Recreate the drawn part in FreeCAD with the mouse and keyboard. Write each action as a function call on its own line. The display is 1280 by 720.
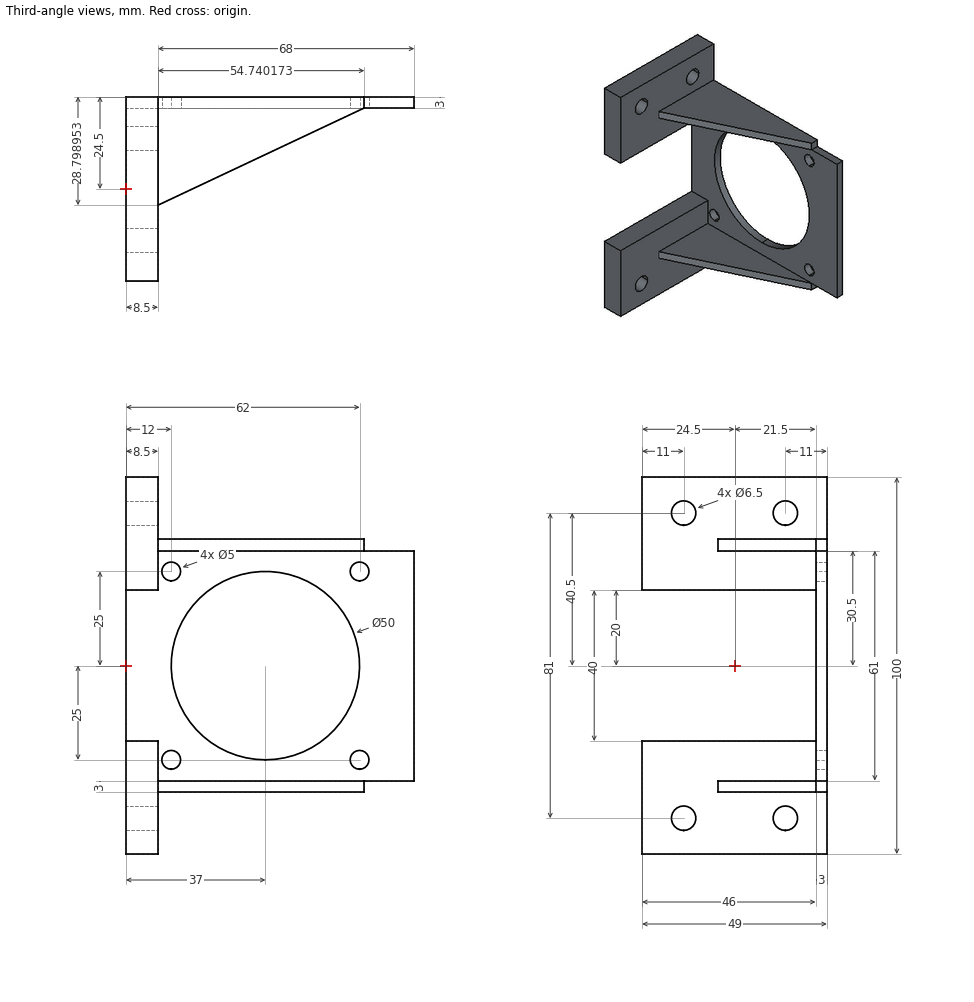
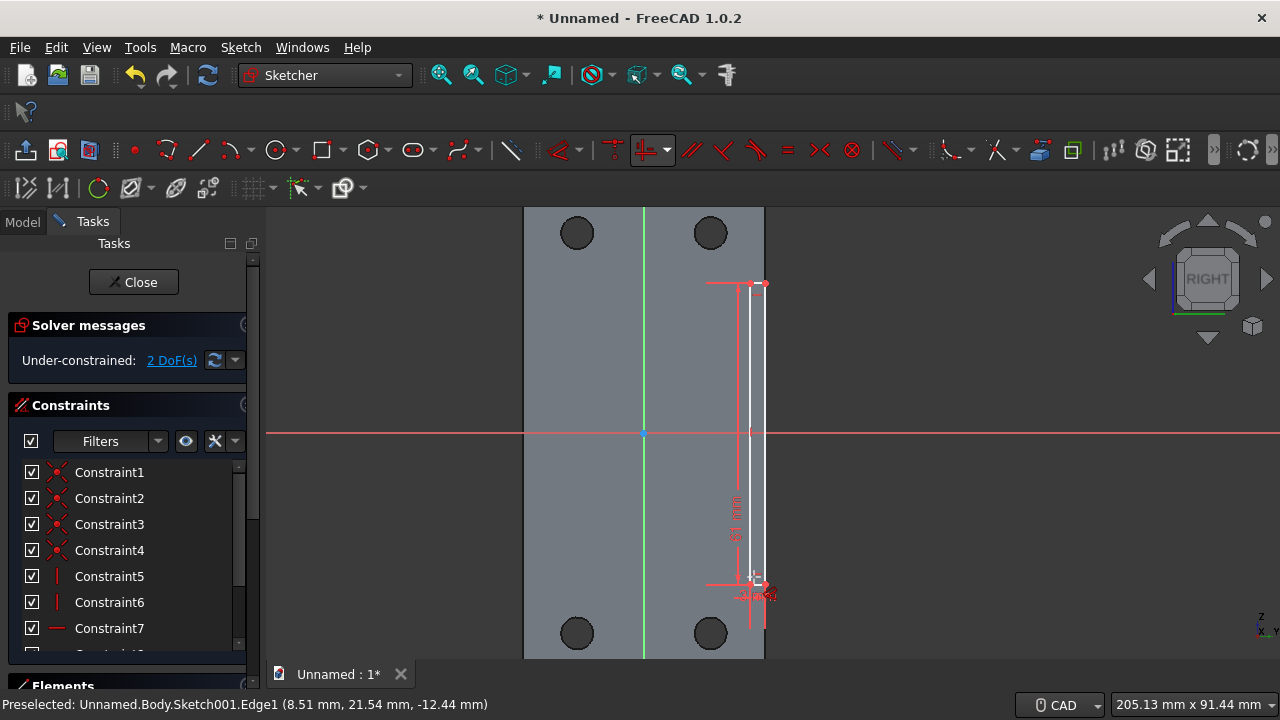
click(750, 283)
click(697, 249)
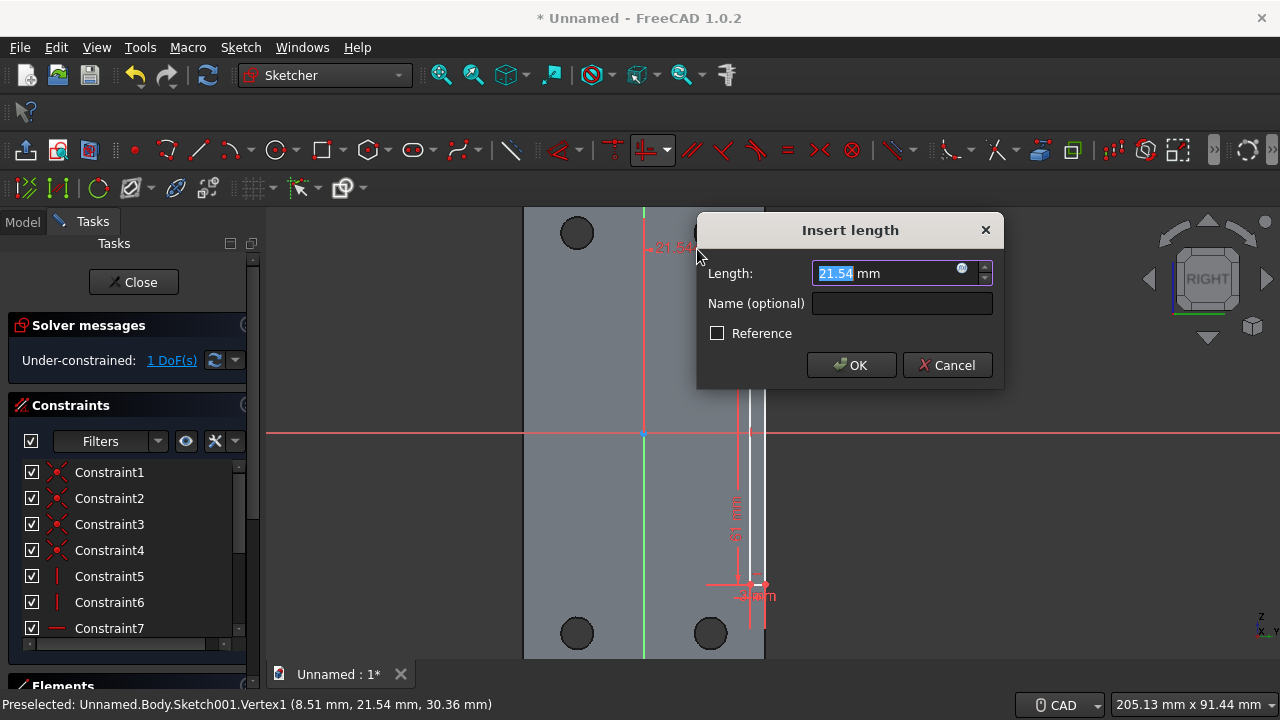
text(21.5)
key(Return)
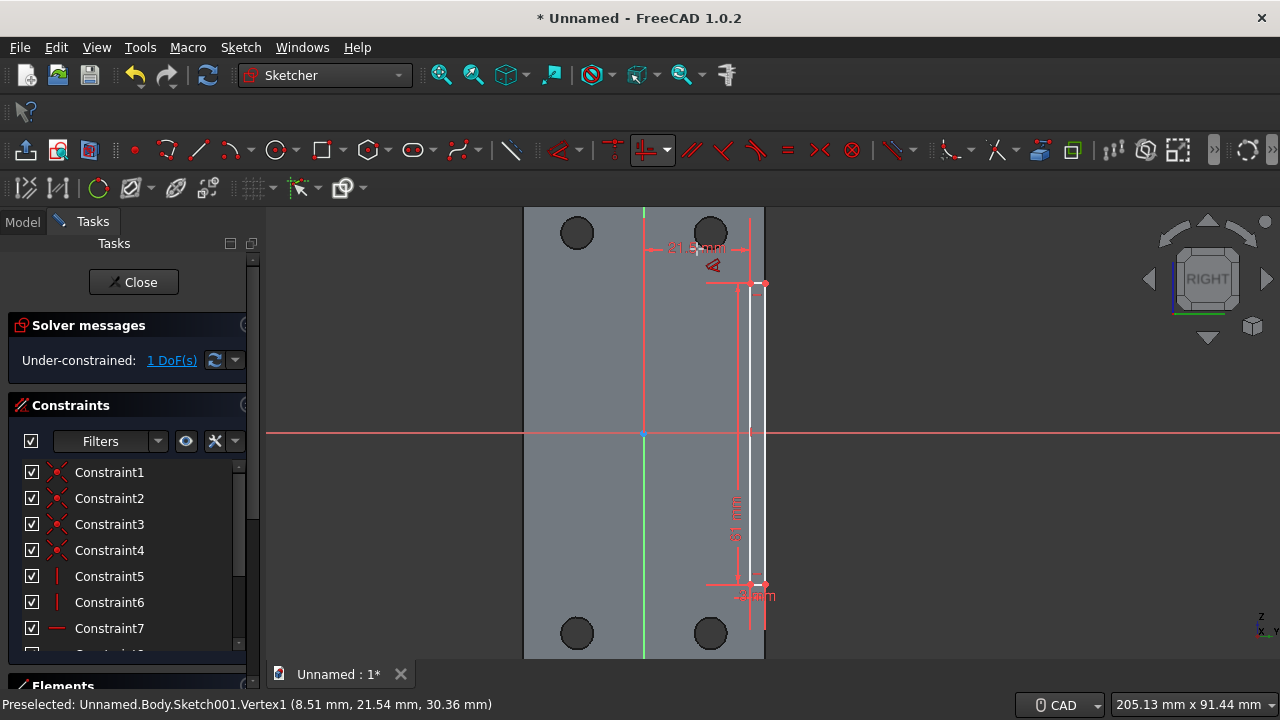
click(750, 283)
click(610, 358)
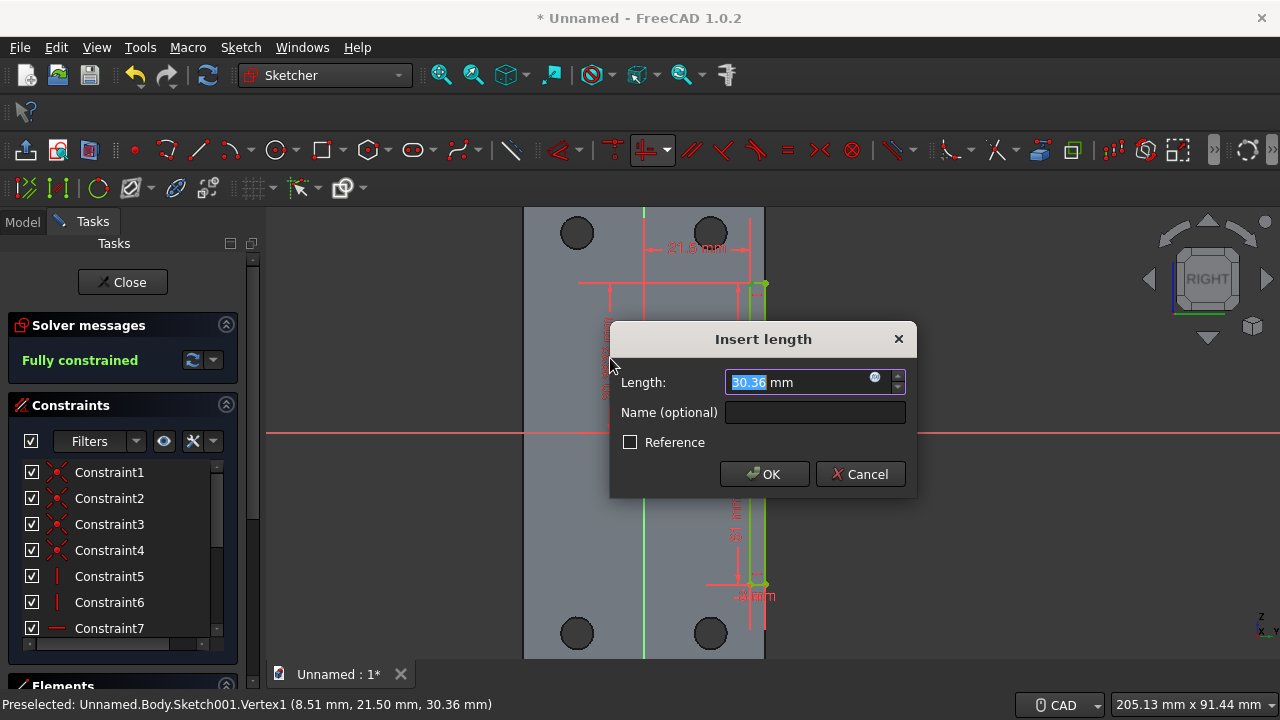
text(30.5)
key(Return)
key(Escape)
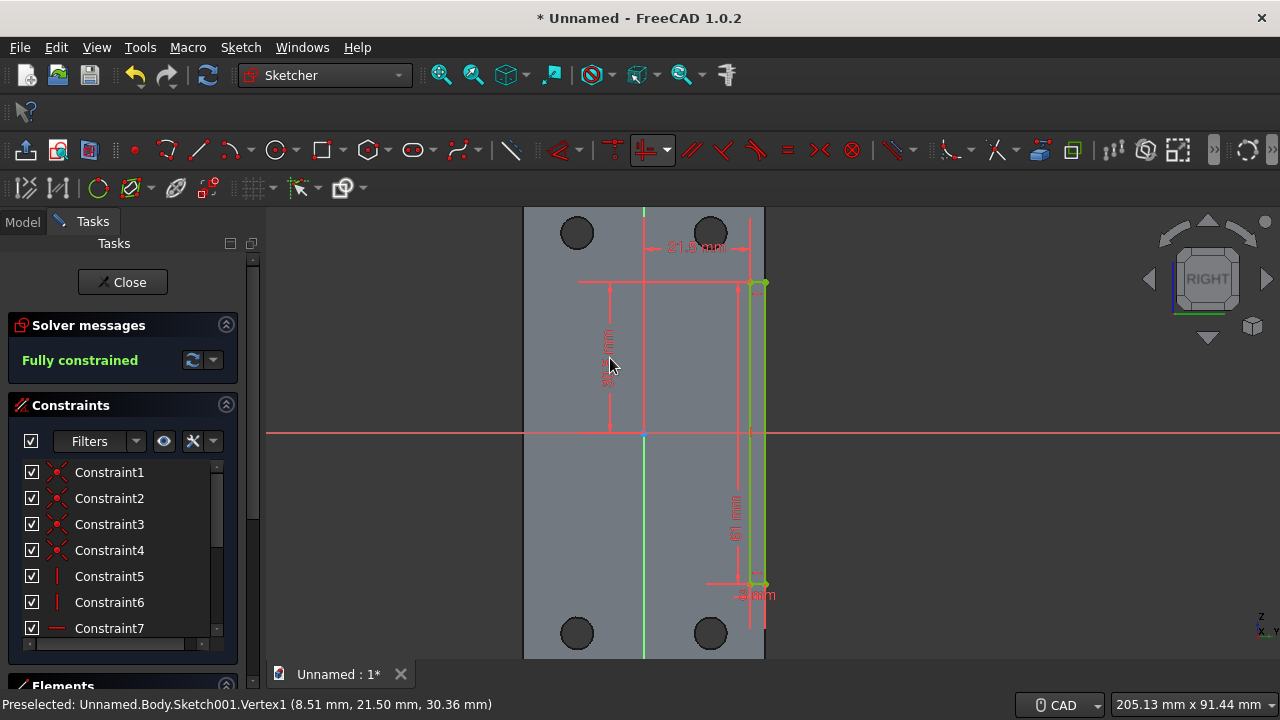
click(123, 282)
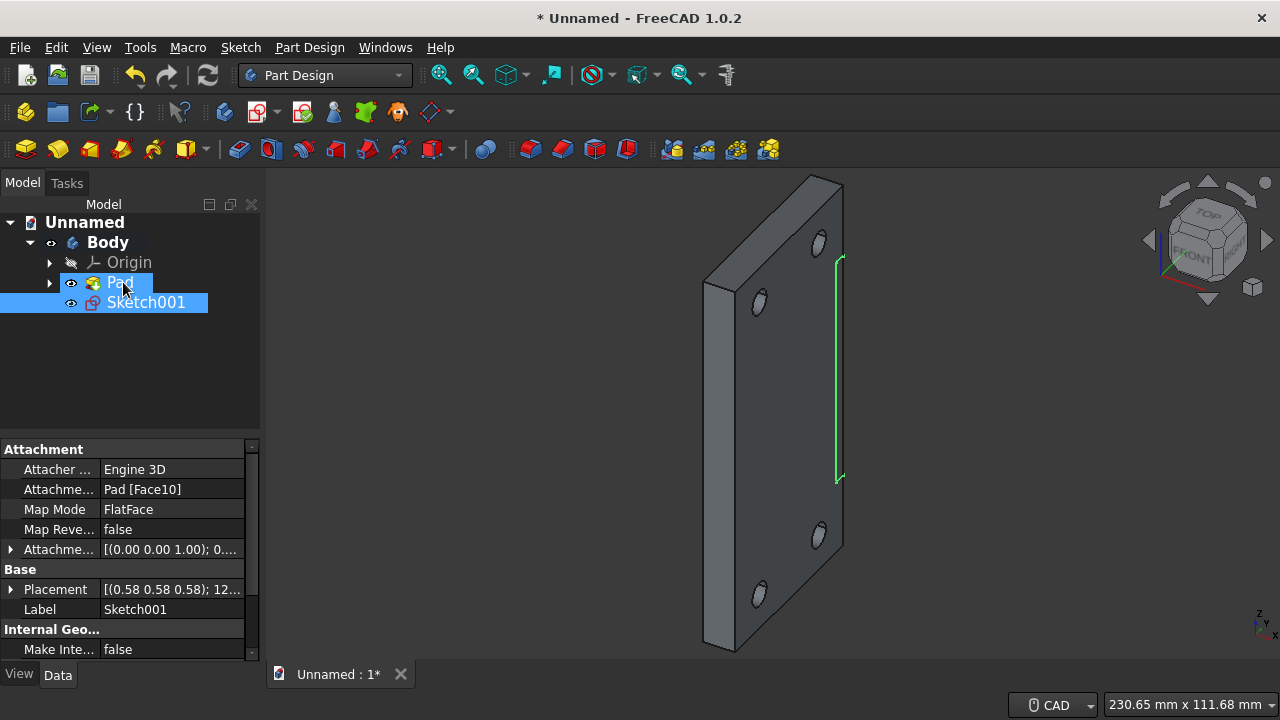
click(26, 150)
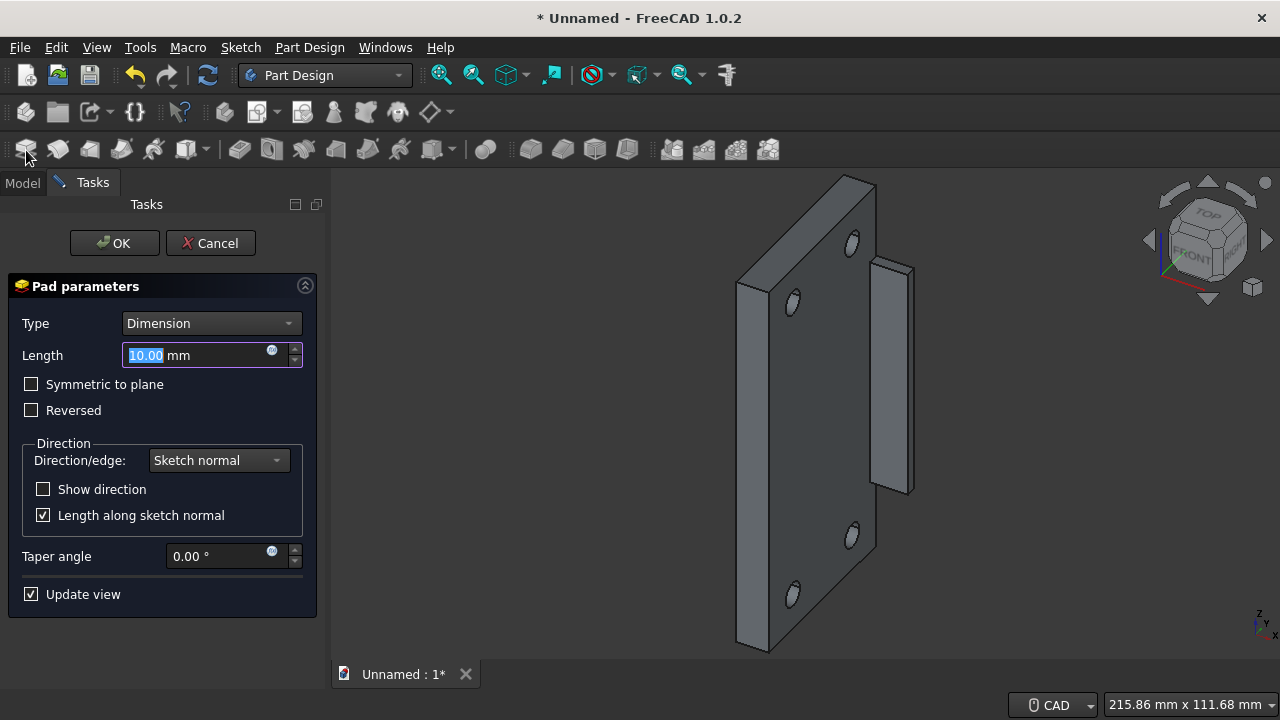
text(68)
key(Tab)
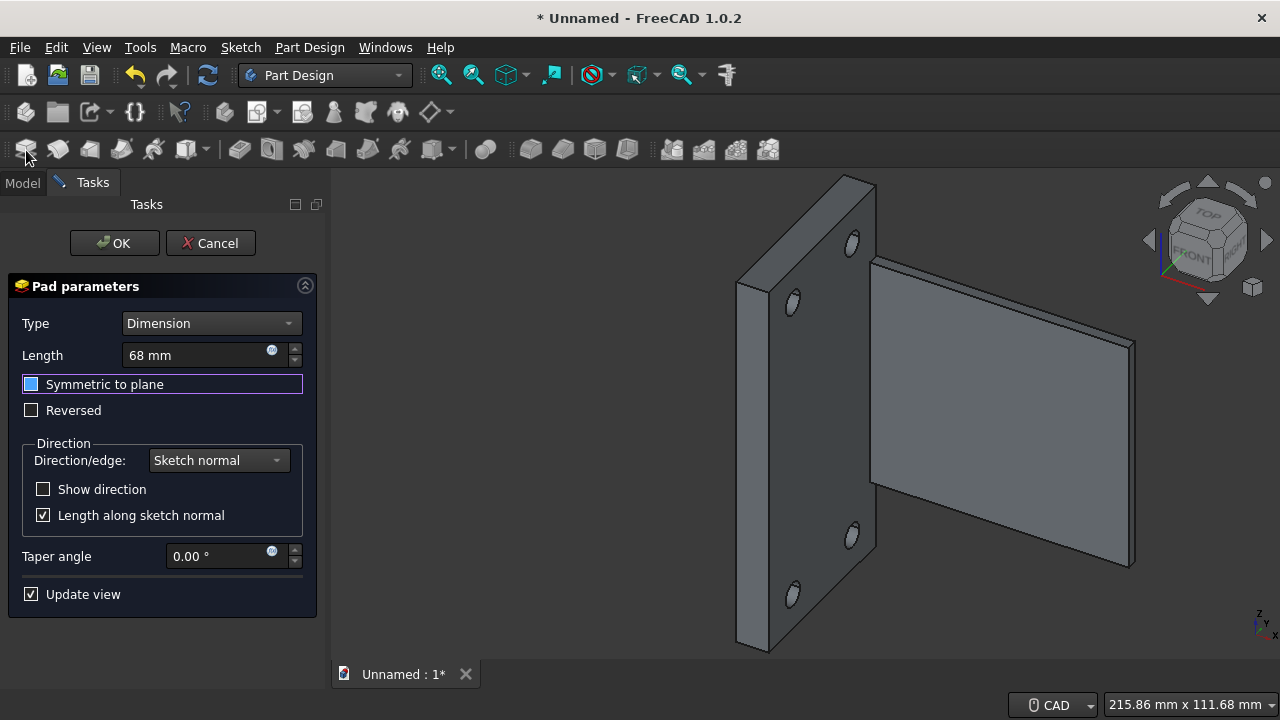
click(115, 243)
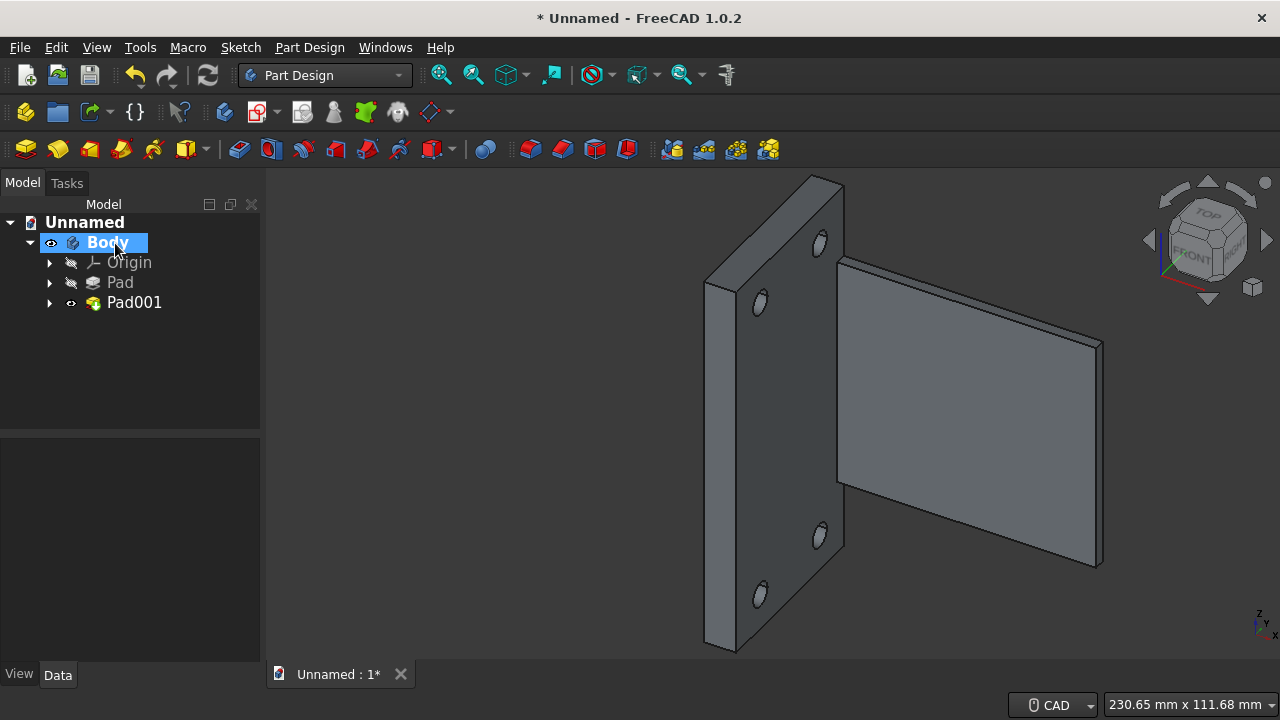
click(442, 76)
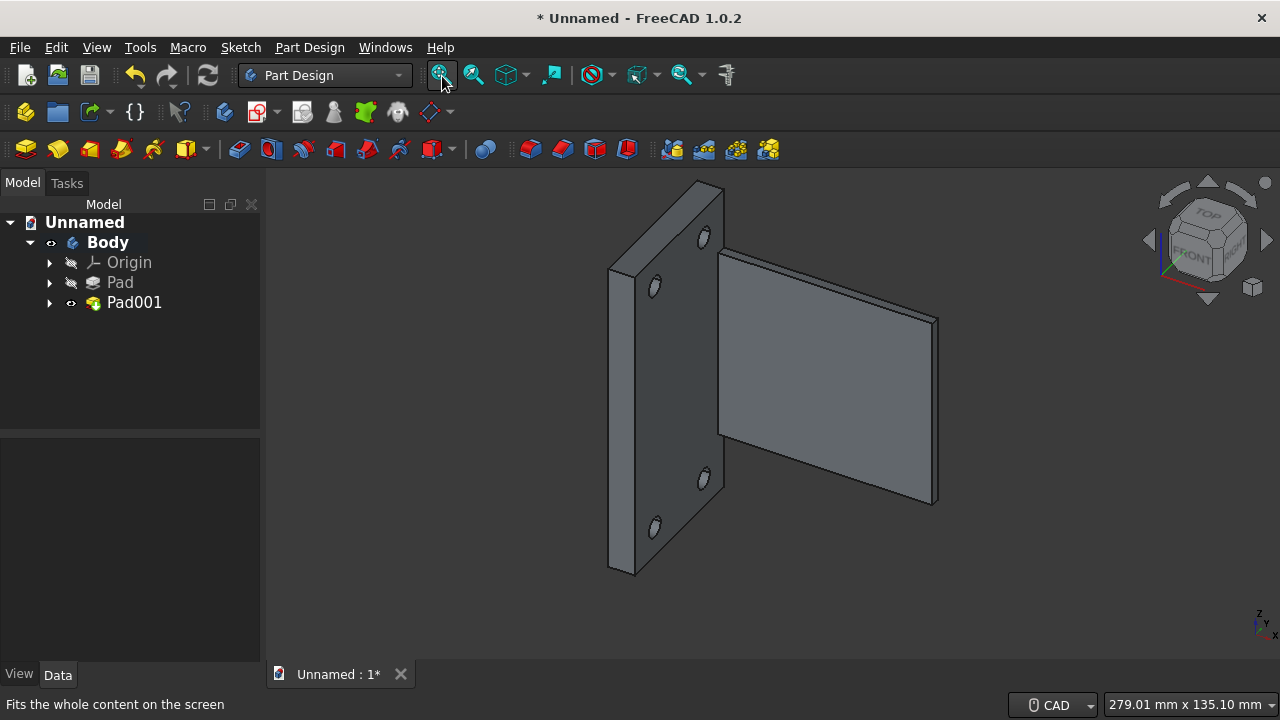
click(825, 378)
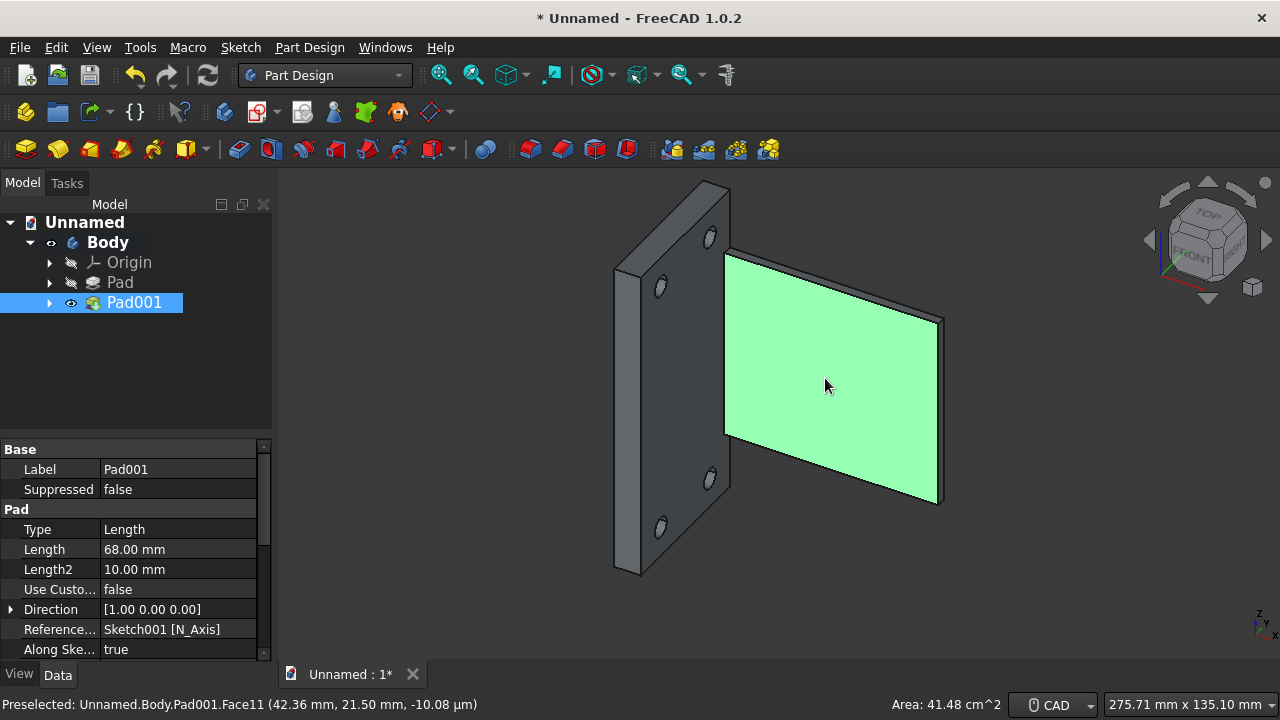
click(258, 112)